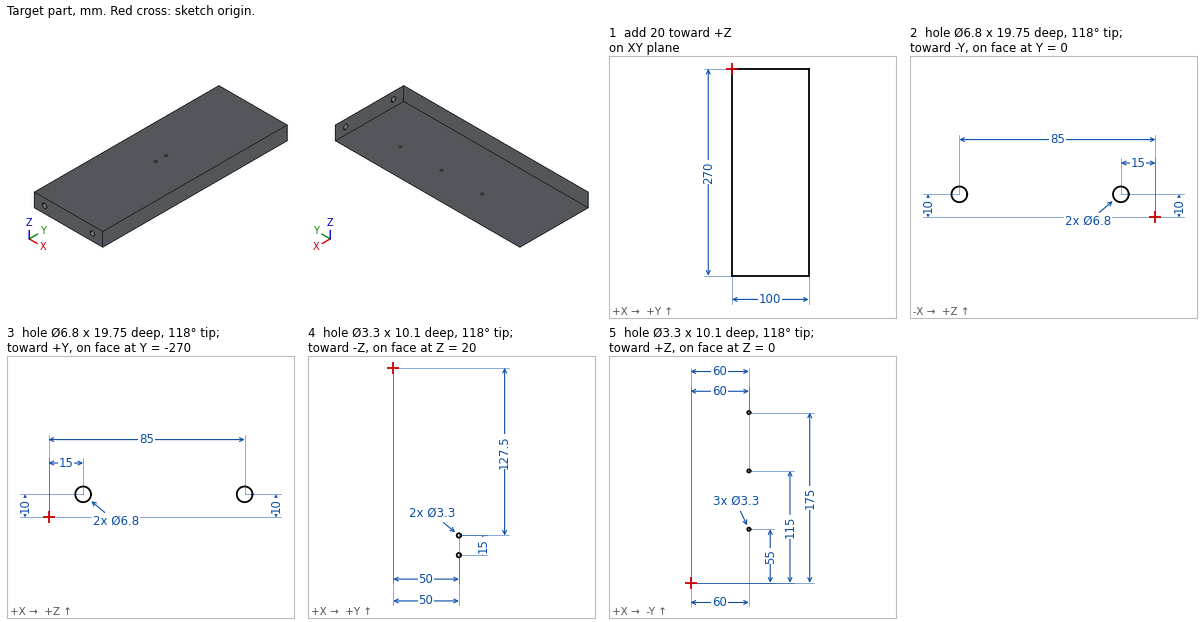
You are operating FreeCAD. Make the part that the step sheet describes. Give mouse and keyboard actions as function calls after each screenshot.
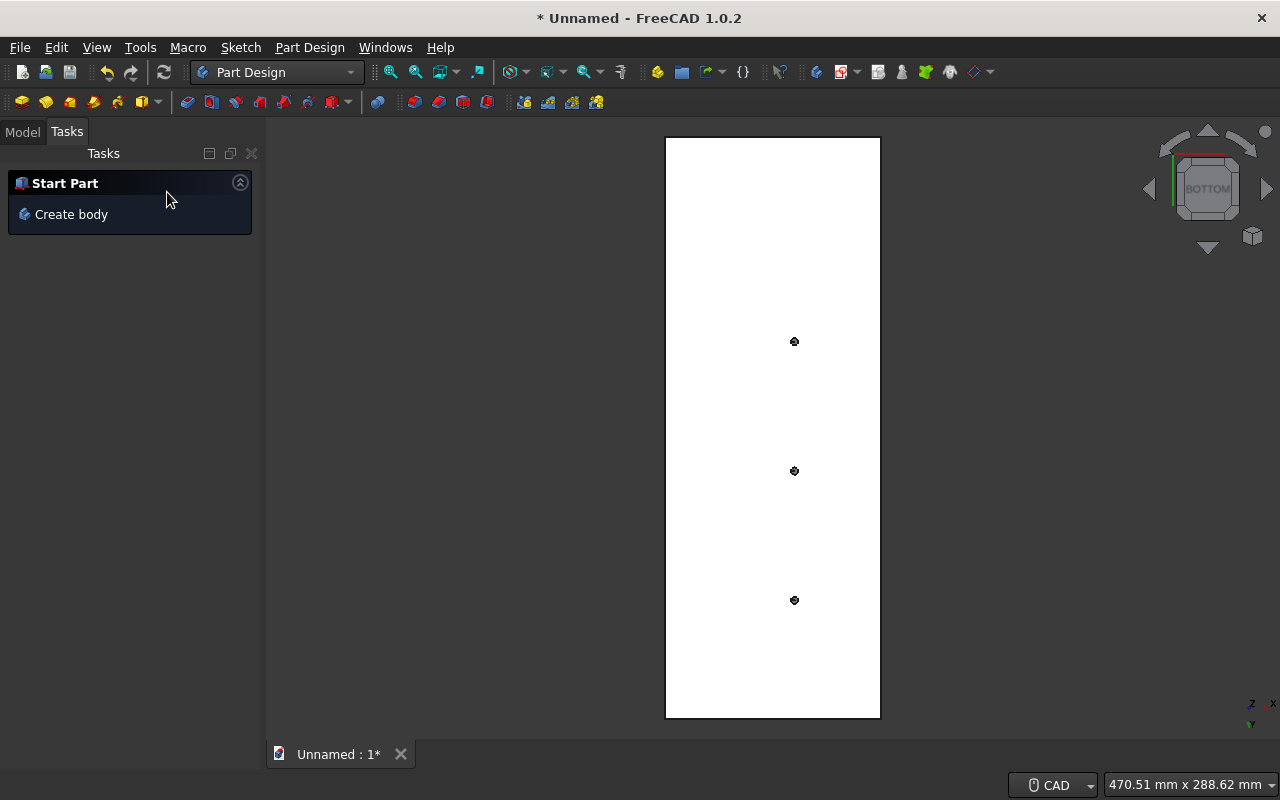
key(0)